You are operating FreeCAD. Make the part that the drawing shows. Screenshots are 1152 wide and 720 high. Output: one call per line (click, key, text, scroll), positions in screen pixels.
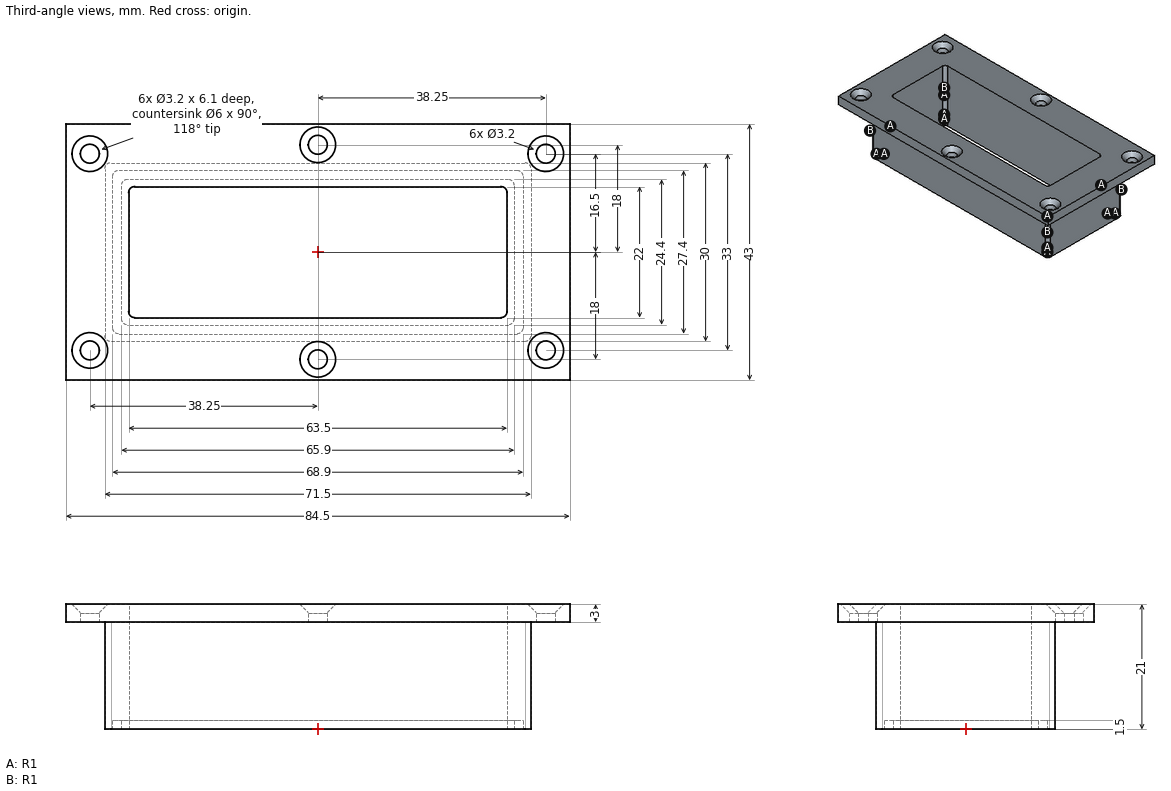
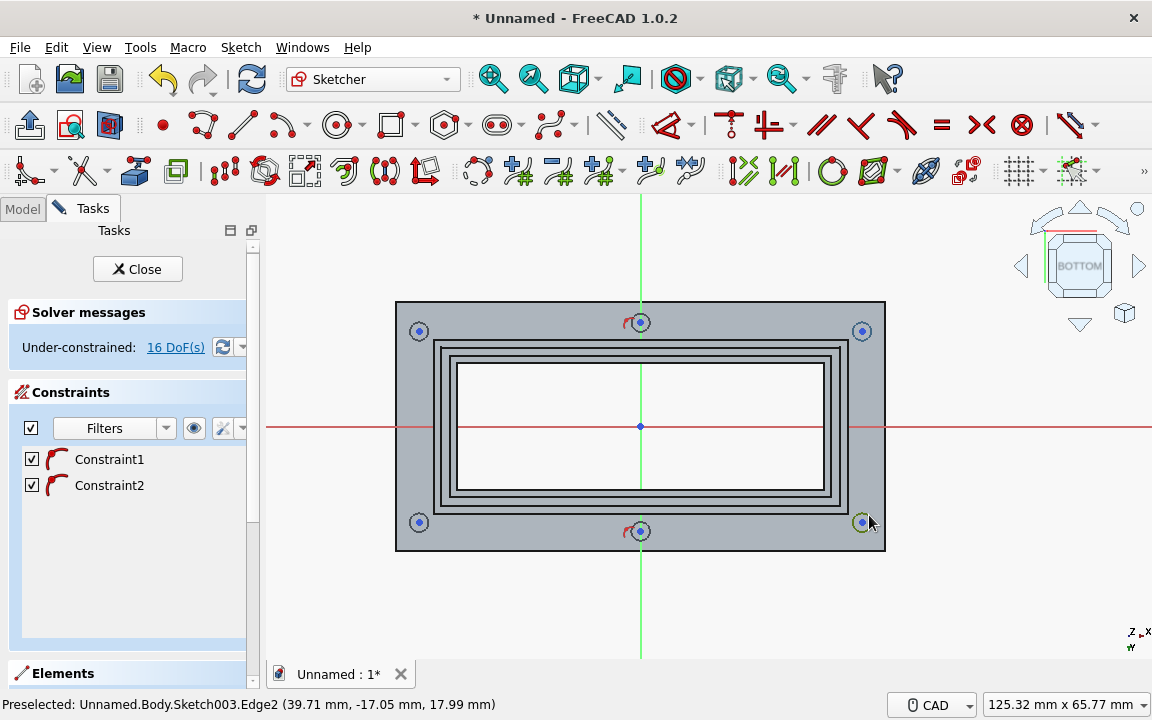
scroll(426, 325, up, 3)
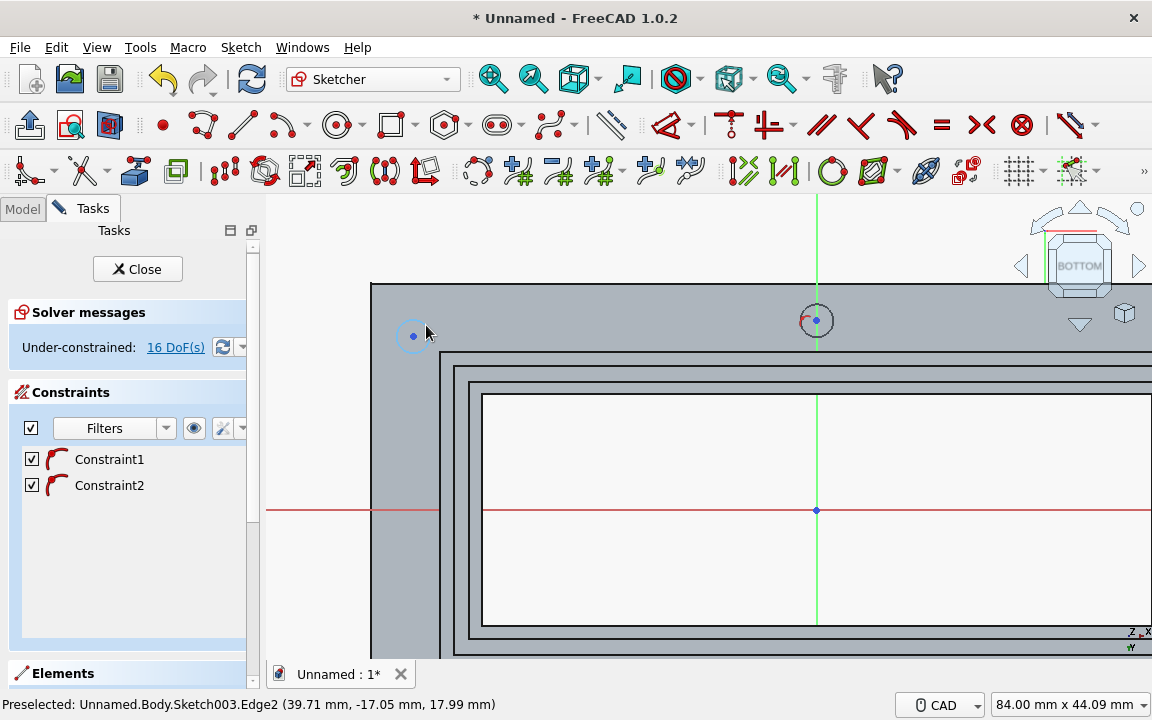
click(425, 325)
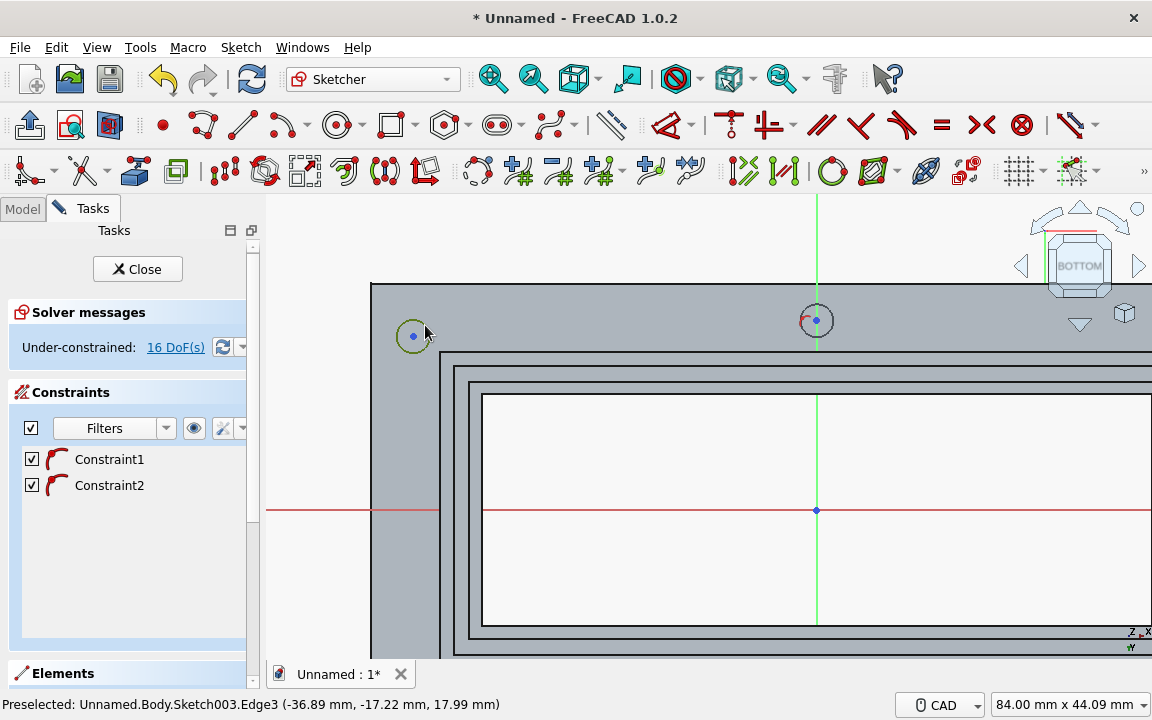
scroll(426, 325, down, 3)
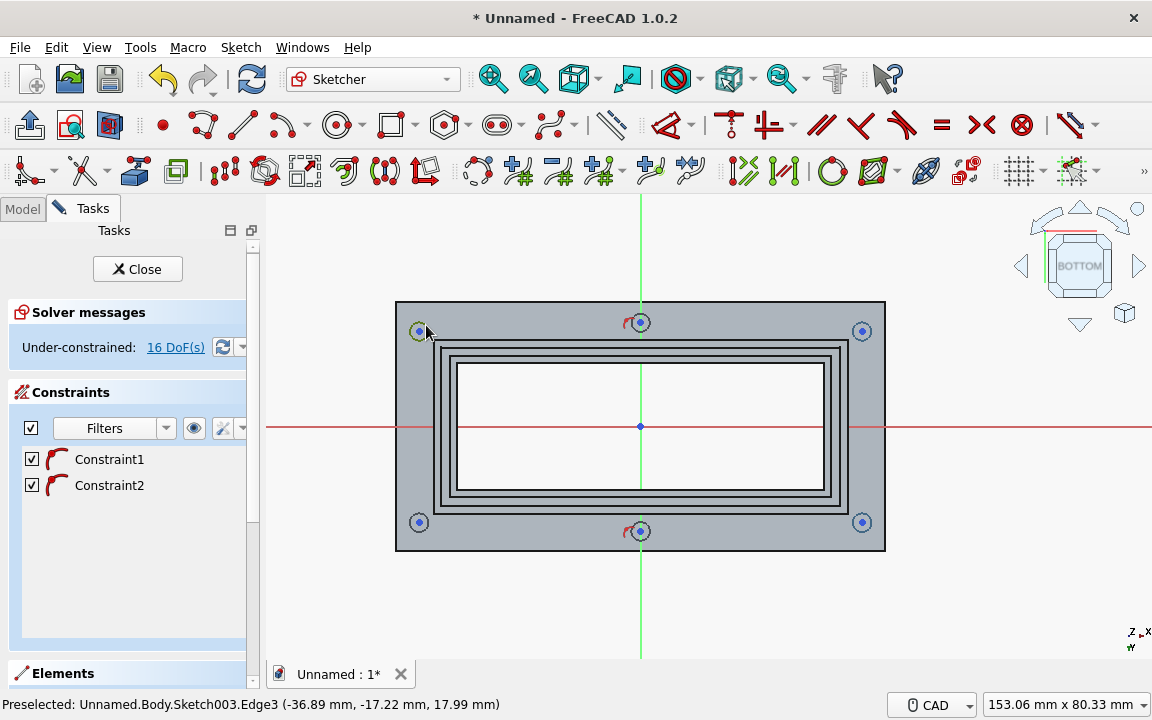
scroll(426, 516, up, 2)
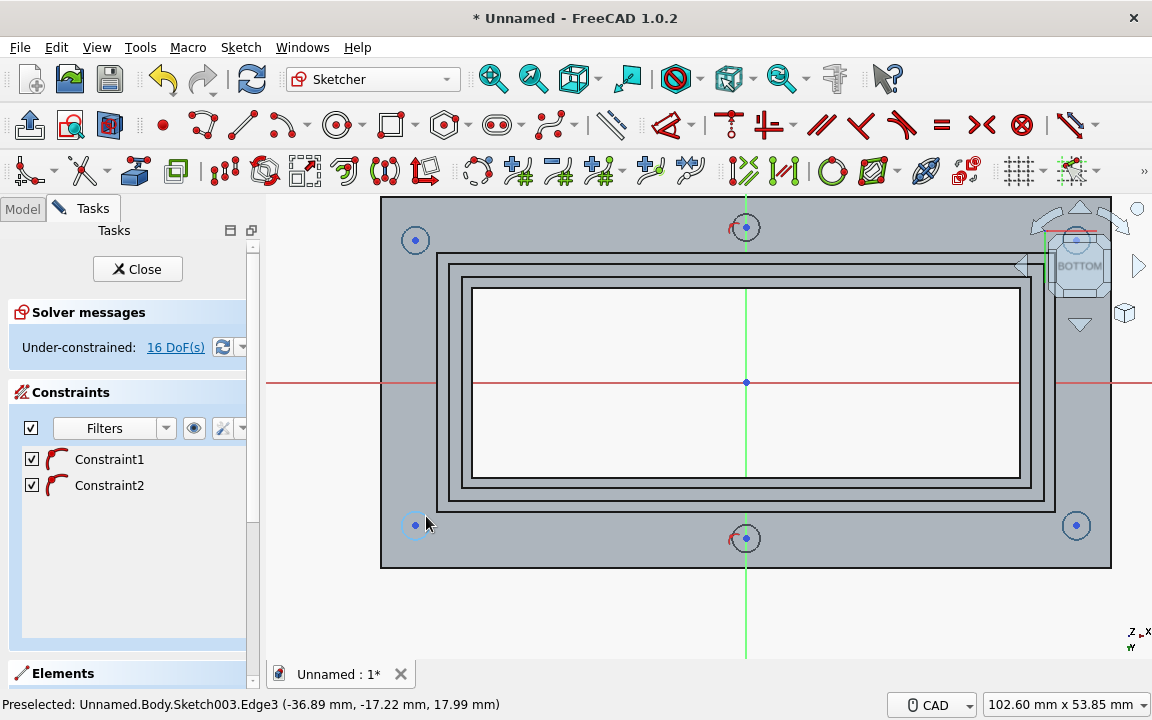
click(425, 516)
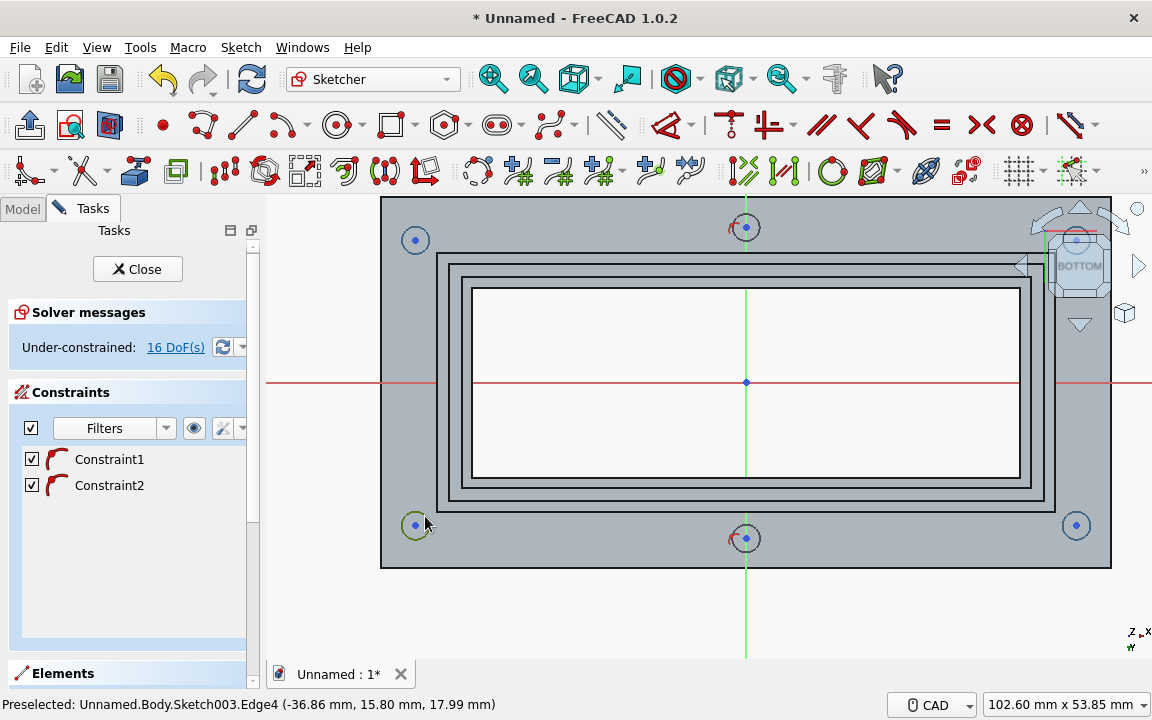
scroll(737, 237, up, 2)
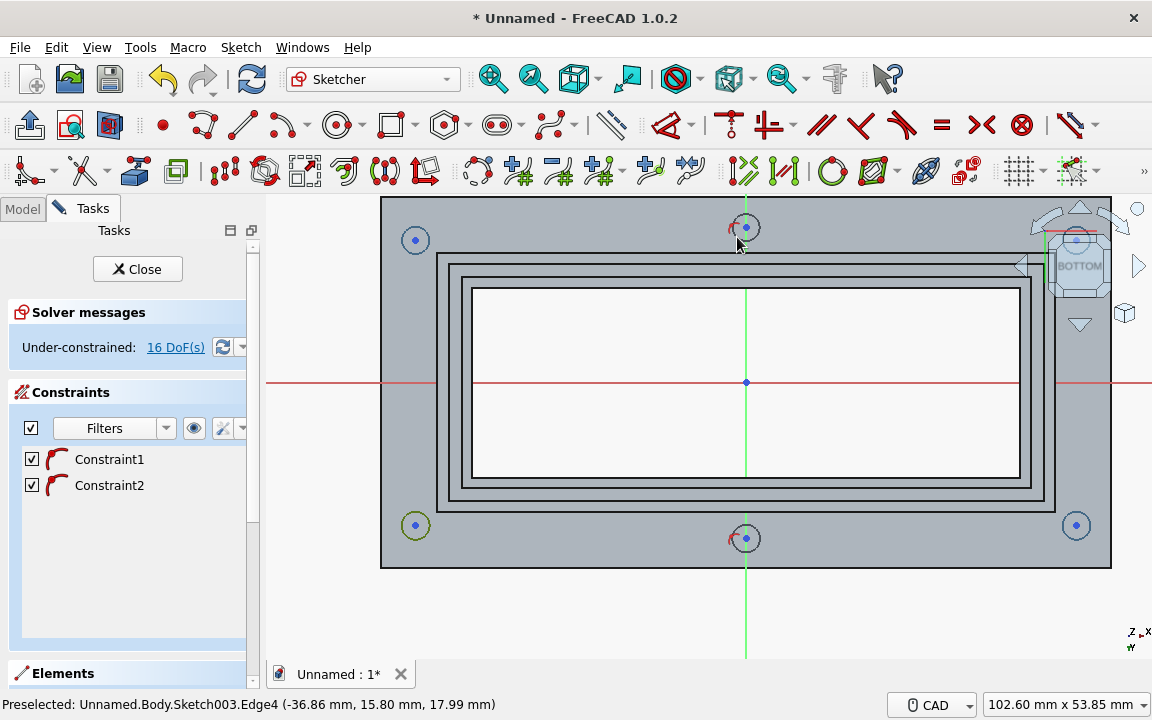
click(736, 237)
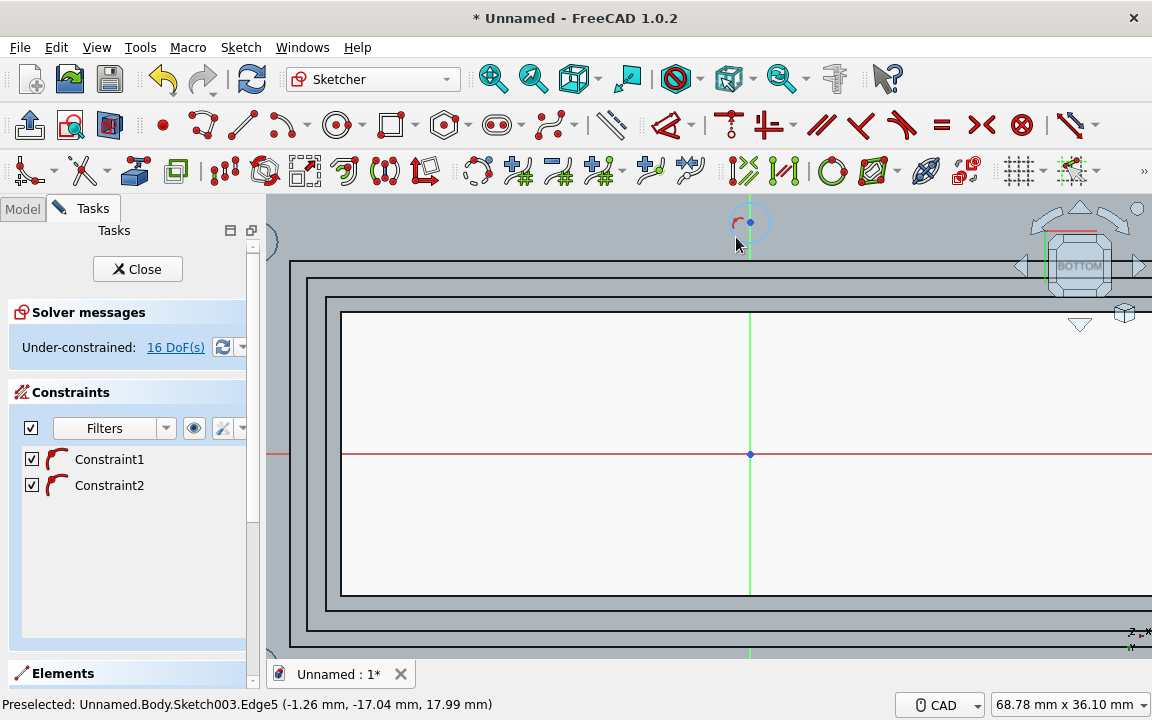
scroll(551, 404, down, 4)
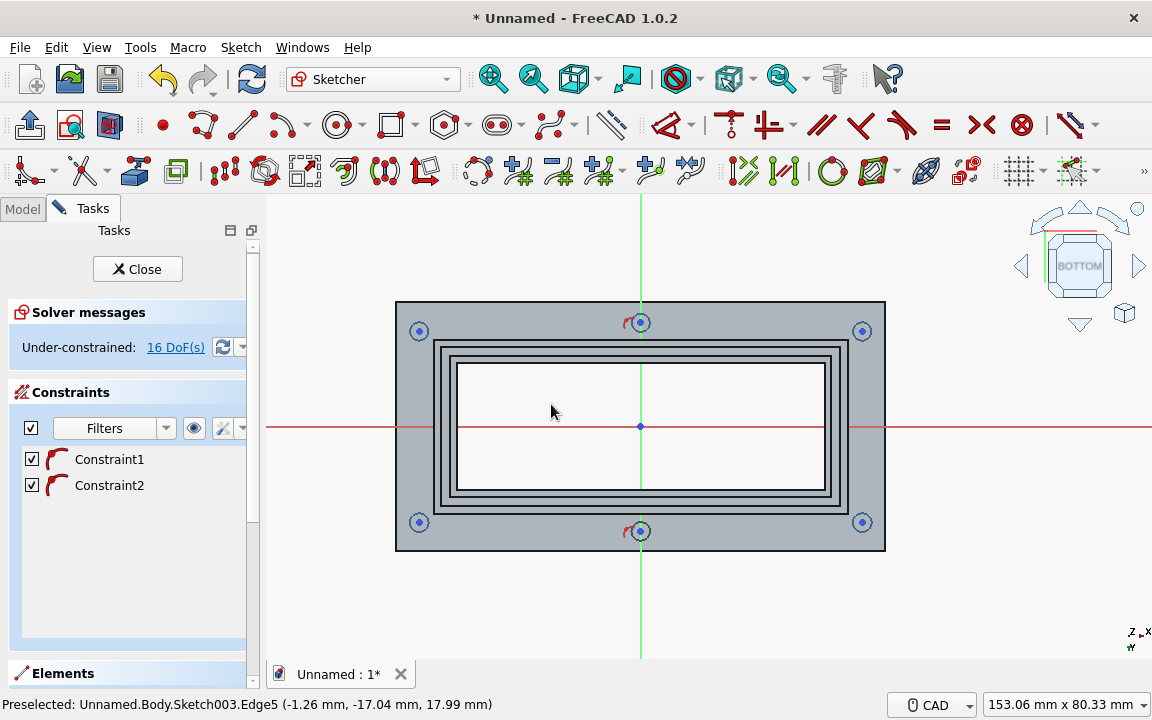
scroll(647, 525, up, 4)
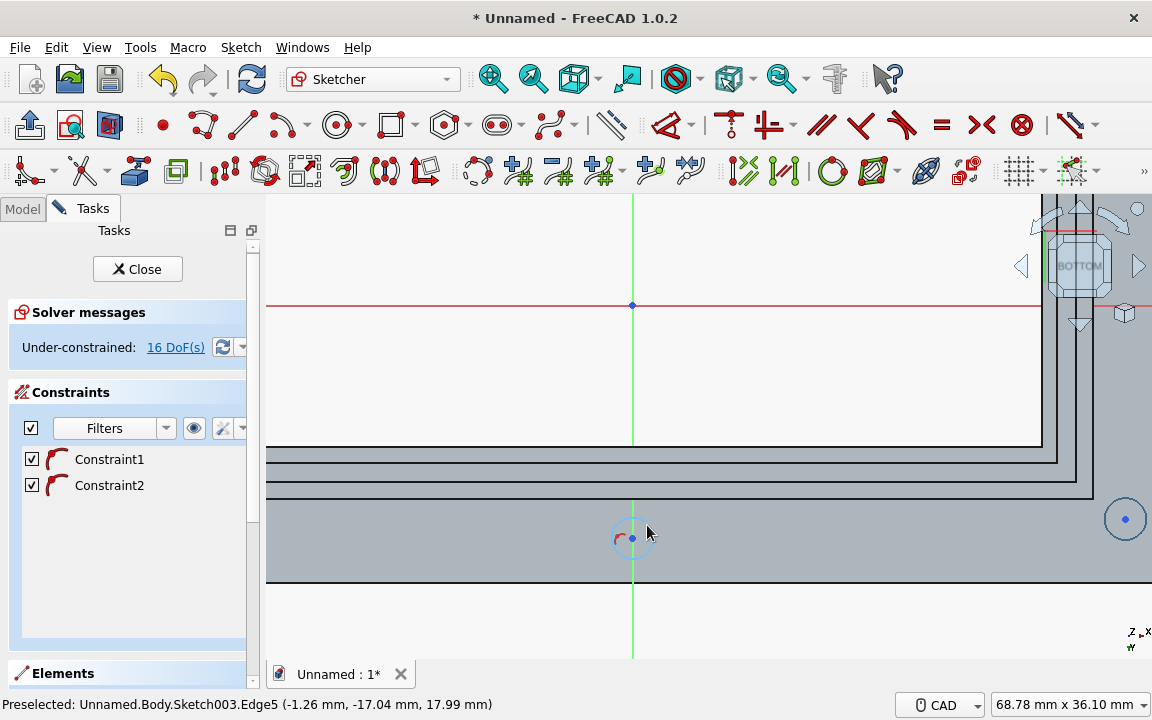
click(647, 524)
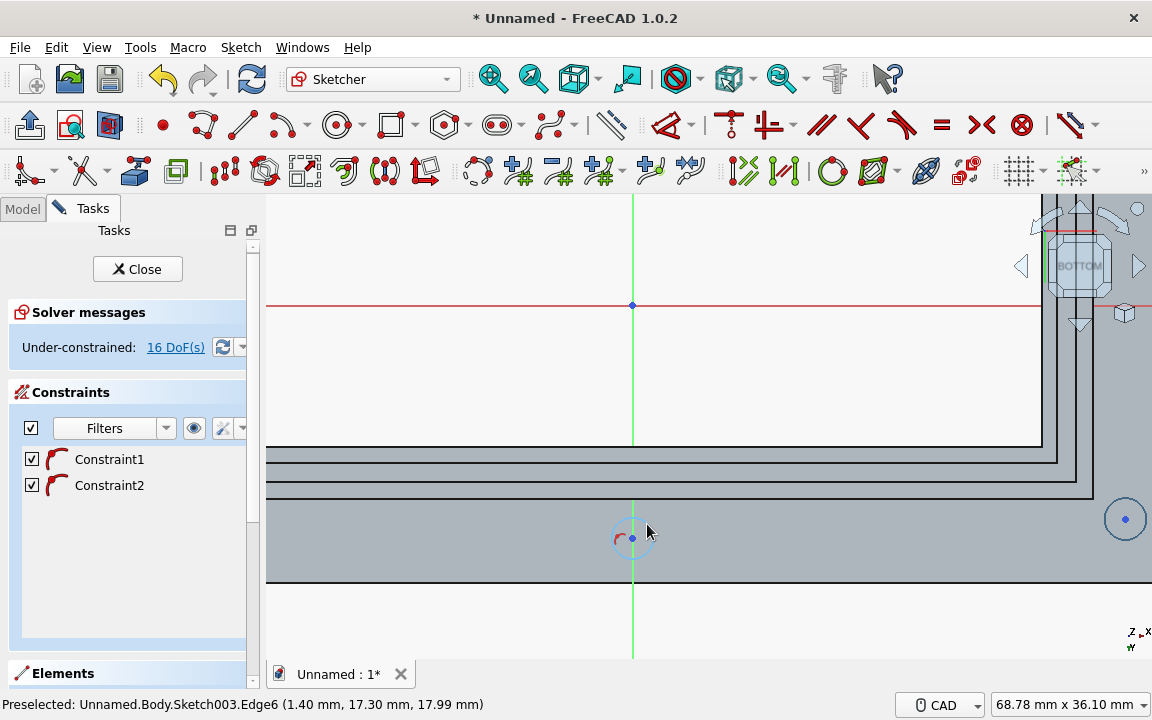
click(942, 126)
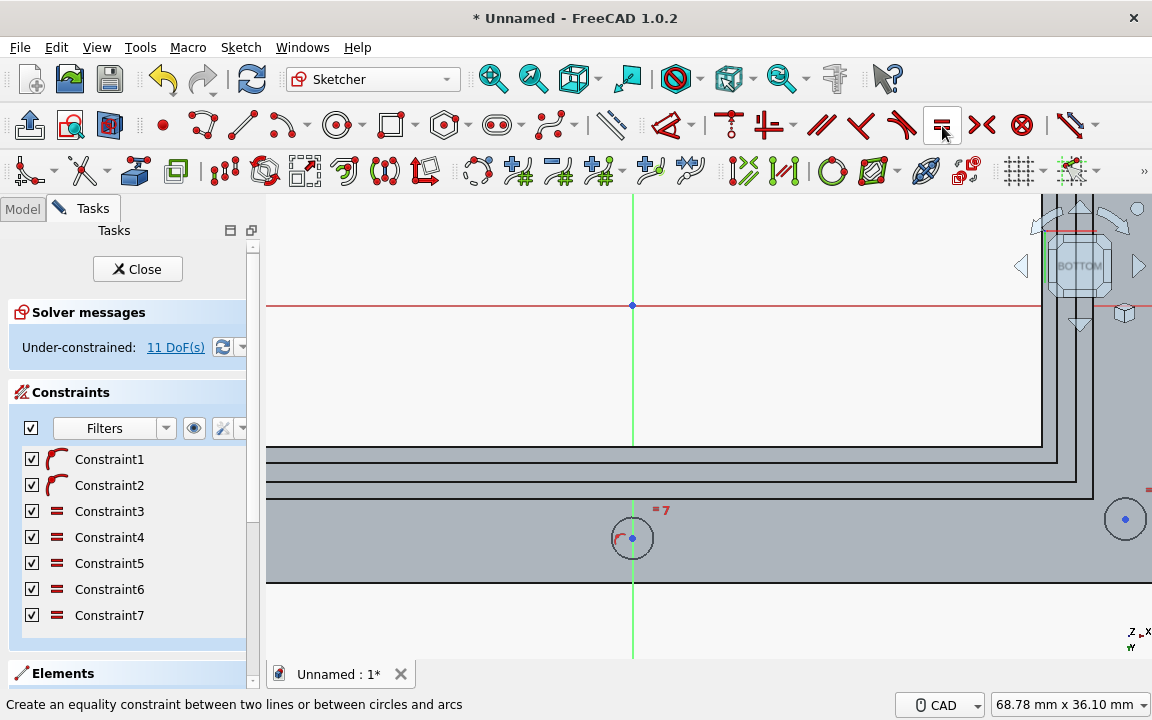
click(666, 126)